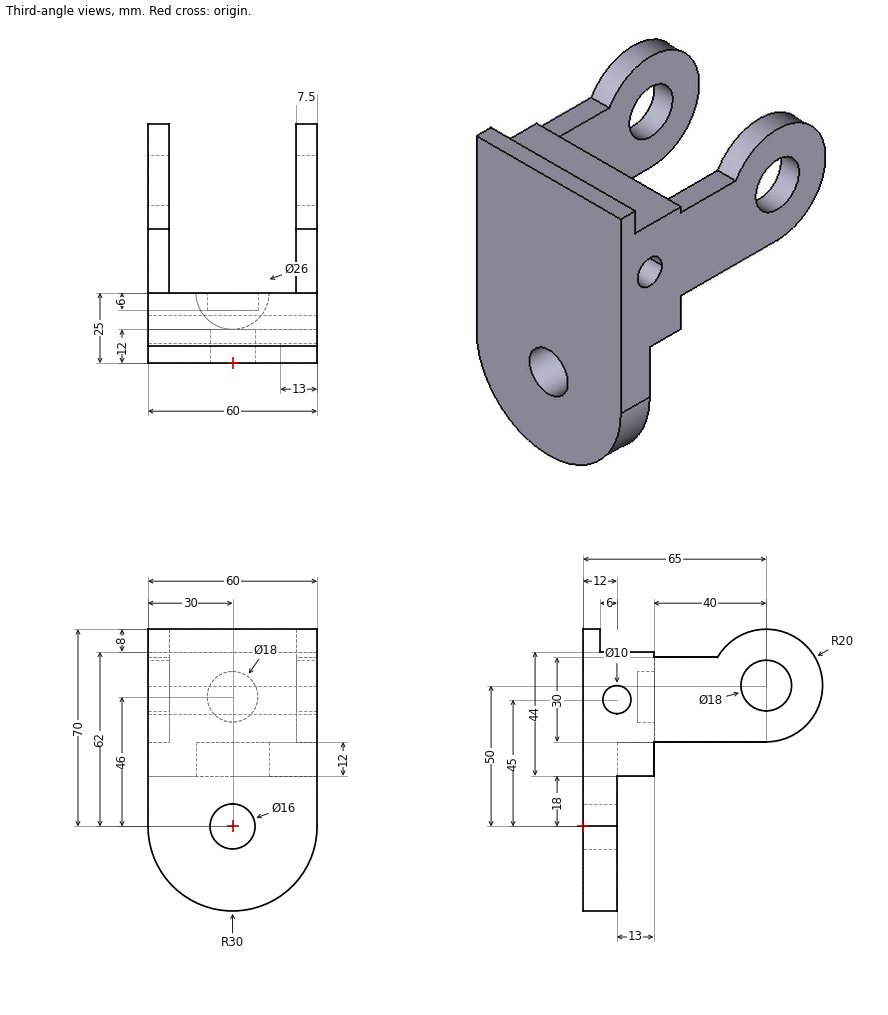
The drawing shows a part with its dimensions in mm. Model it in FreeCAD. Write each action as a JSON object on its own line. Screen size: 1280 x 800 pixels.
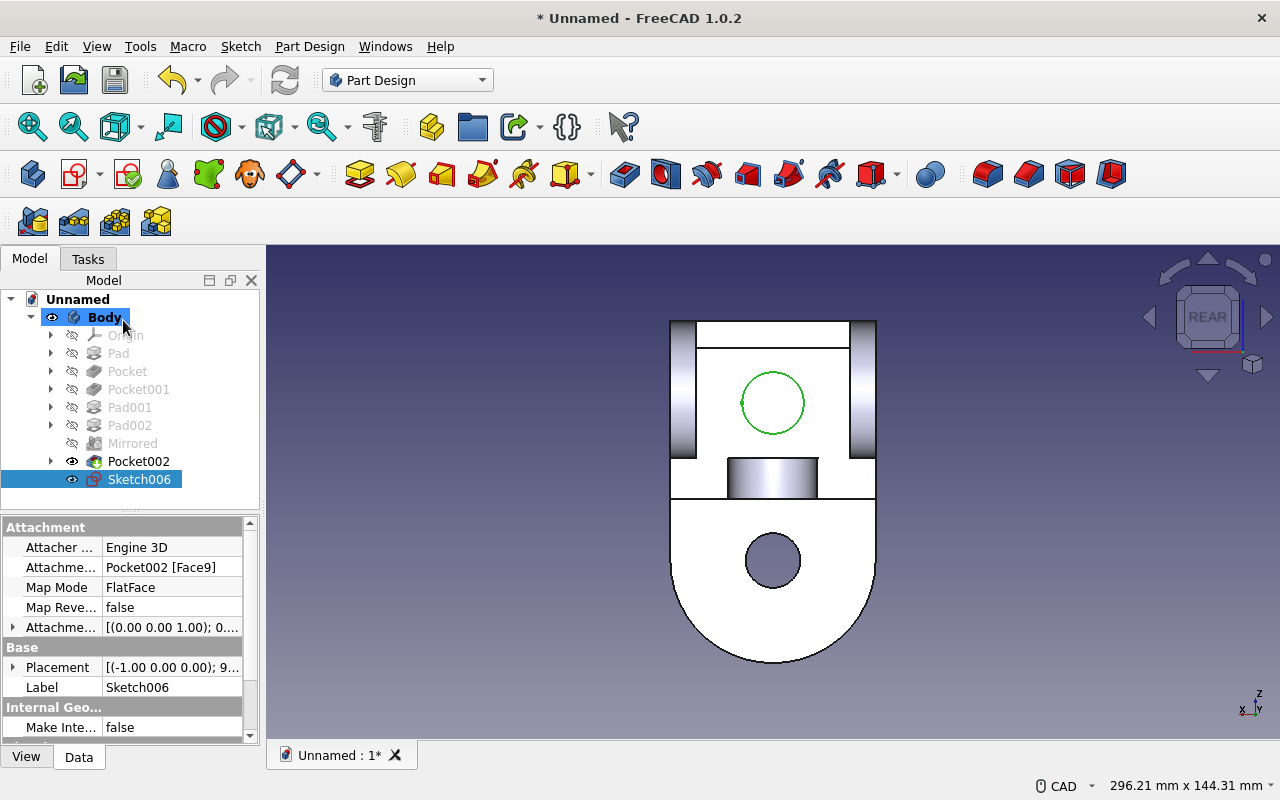
{"action": "left_click", "coordinate": [625, 174]}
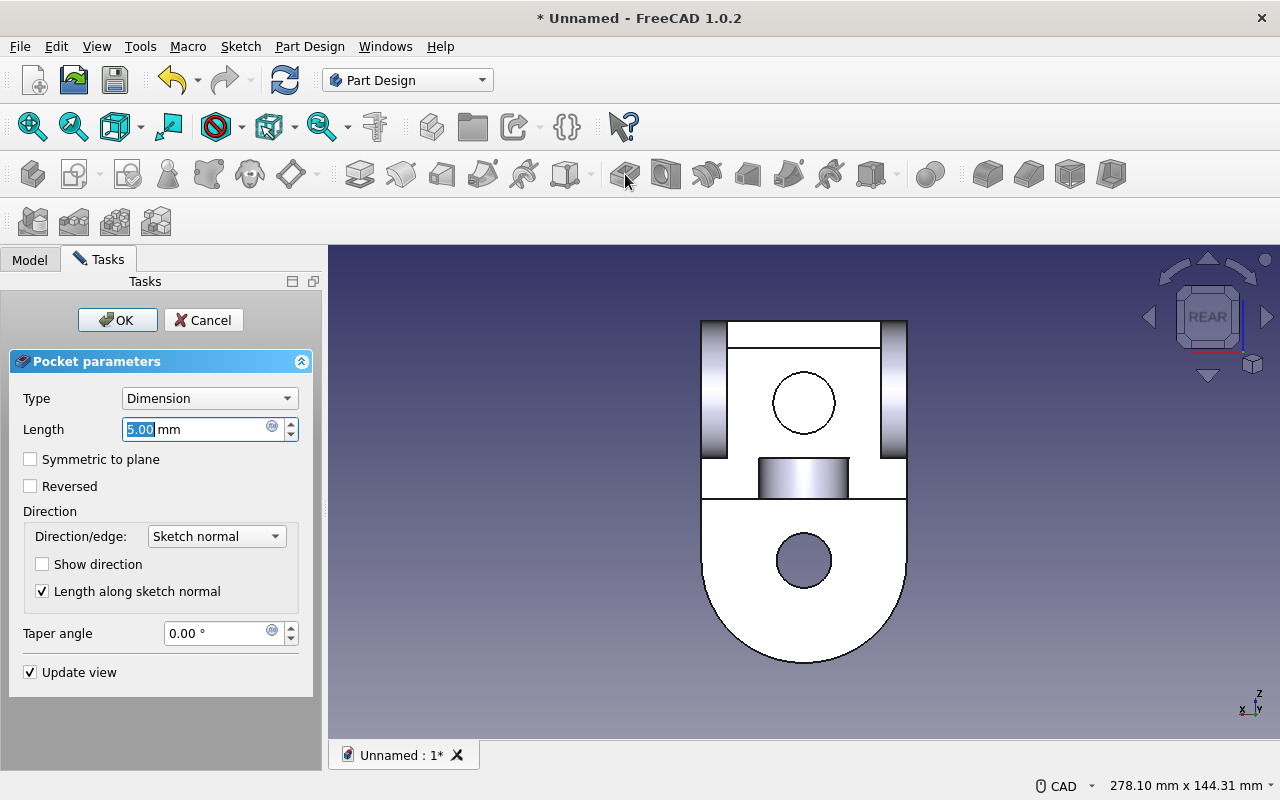
{"action": "type", "text": "6"}
{"action": "key", "text": "Tab"}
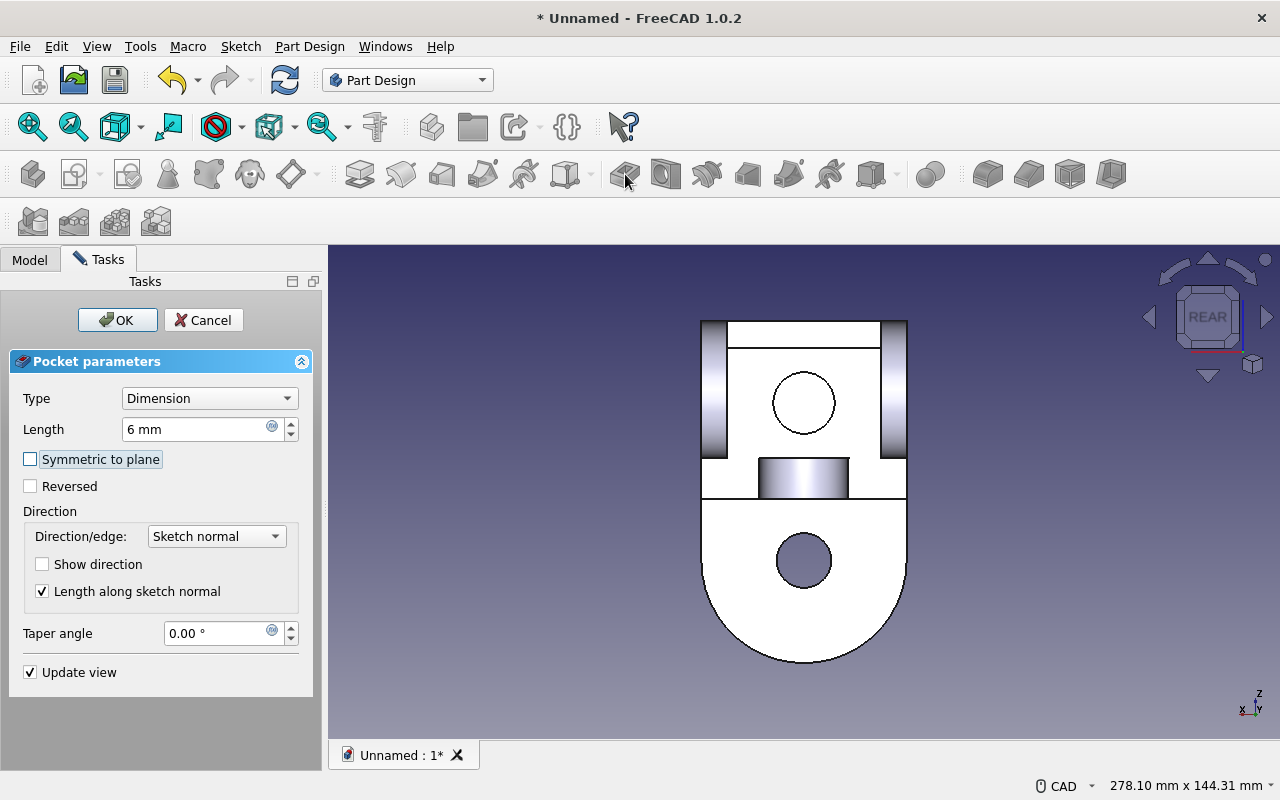
{"action": "left_click", "coordinate": [118, 320]}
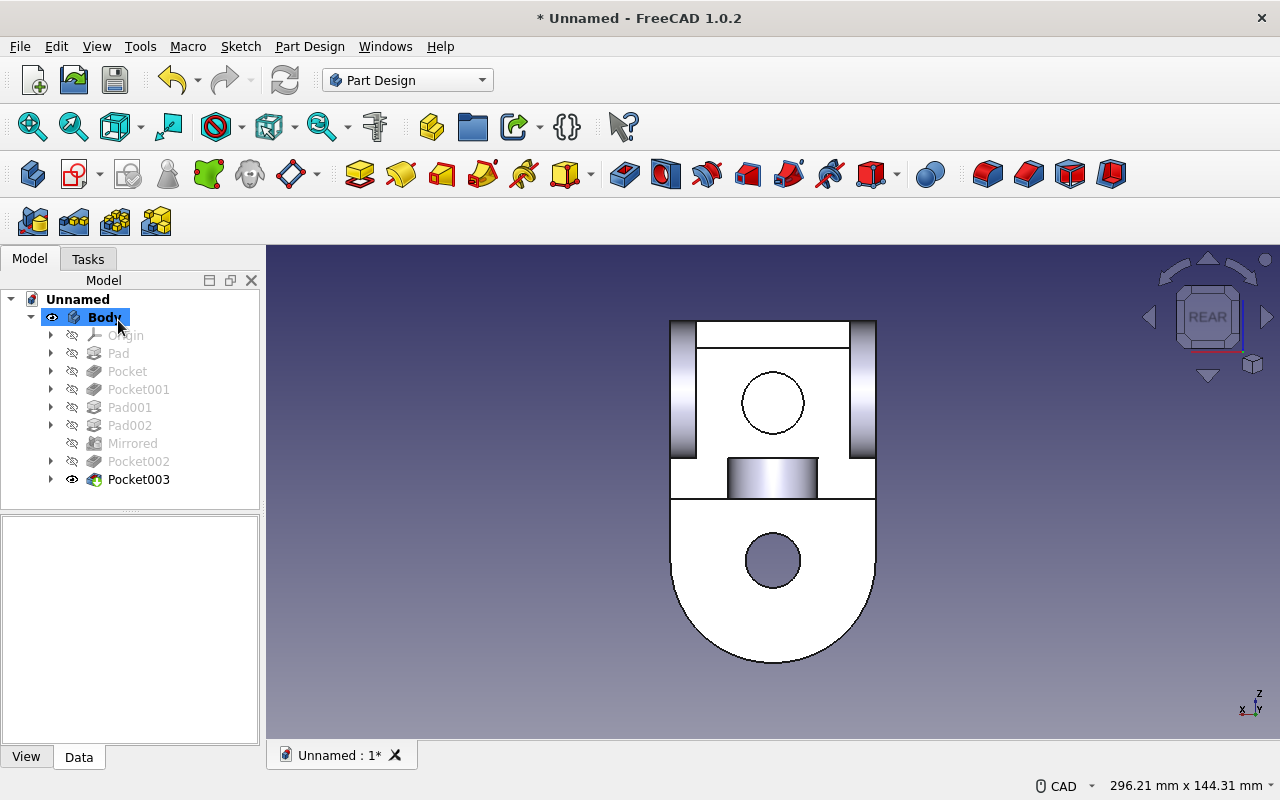
{"action": "key", "text": "0"}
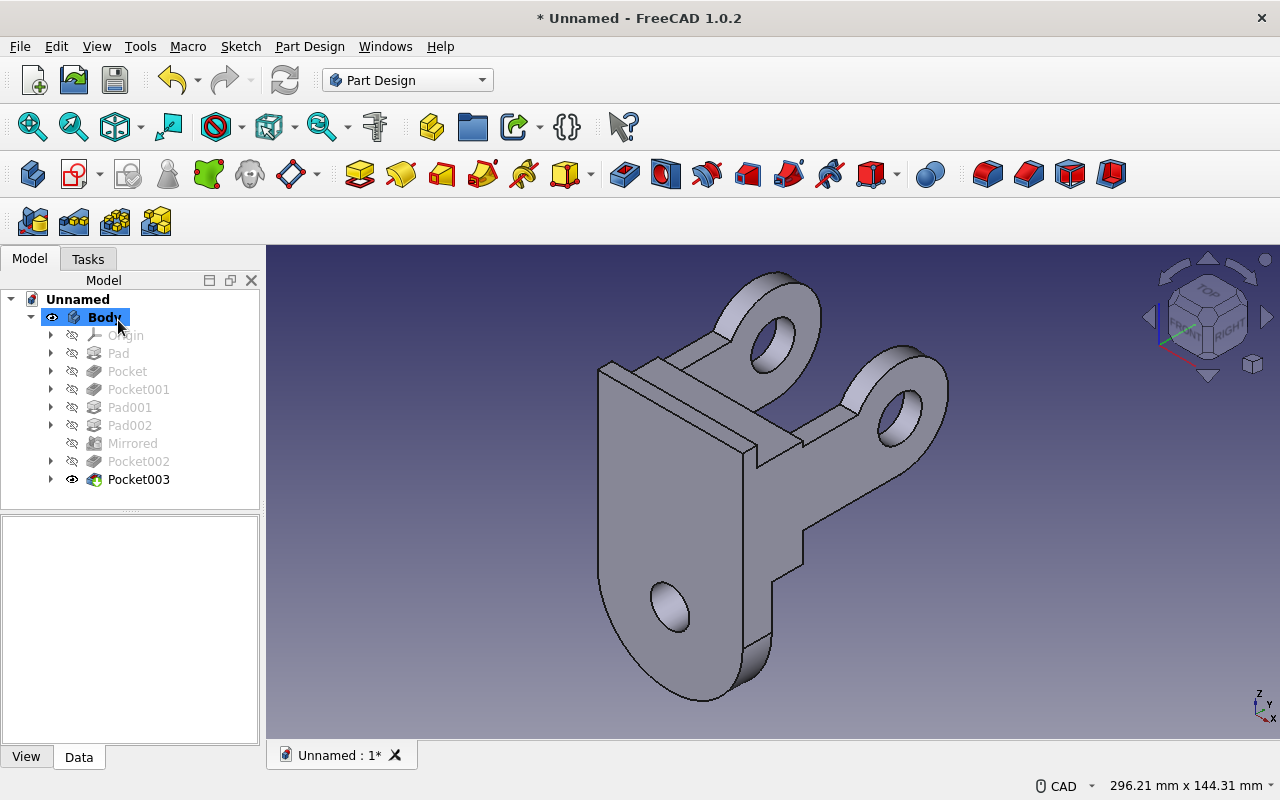
{"action": "left_click", "coordinate": [787, 497]}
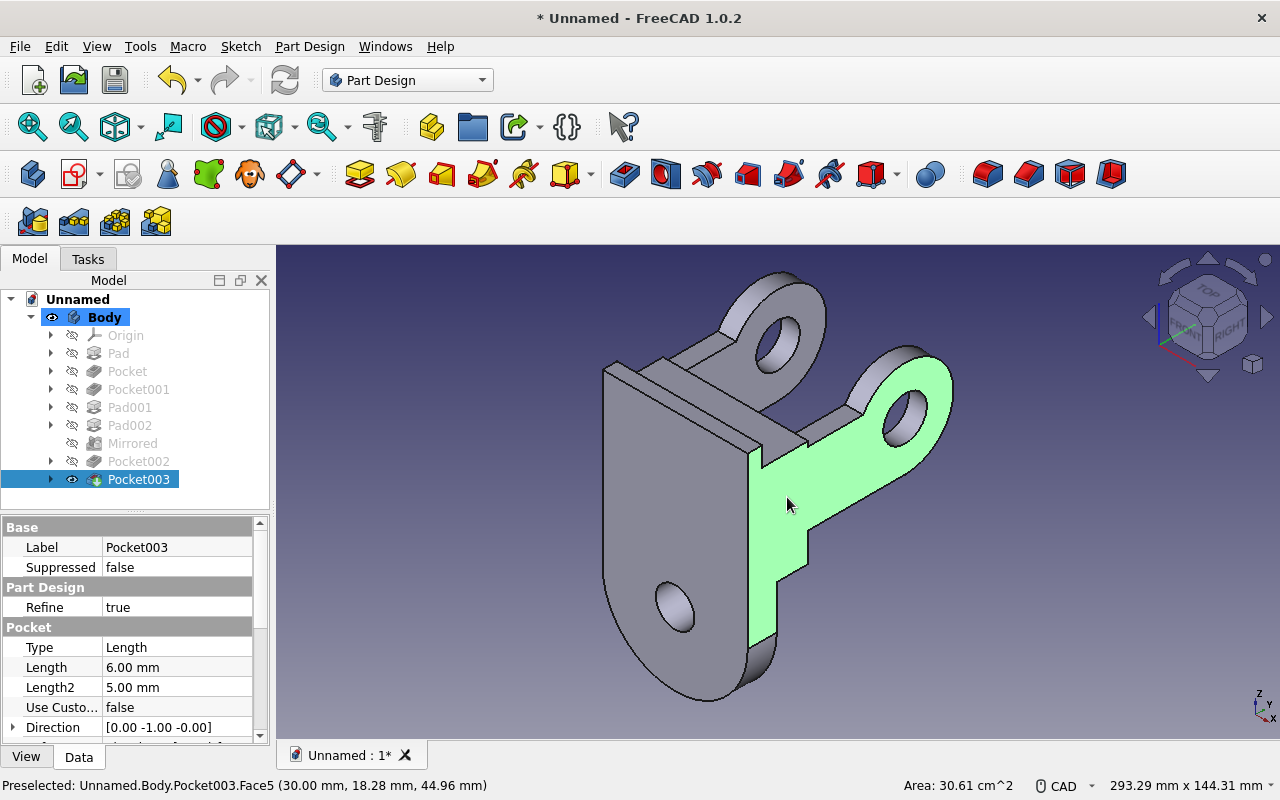
{"action": "left_click", "coordinate": [74, 174]}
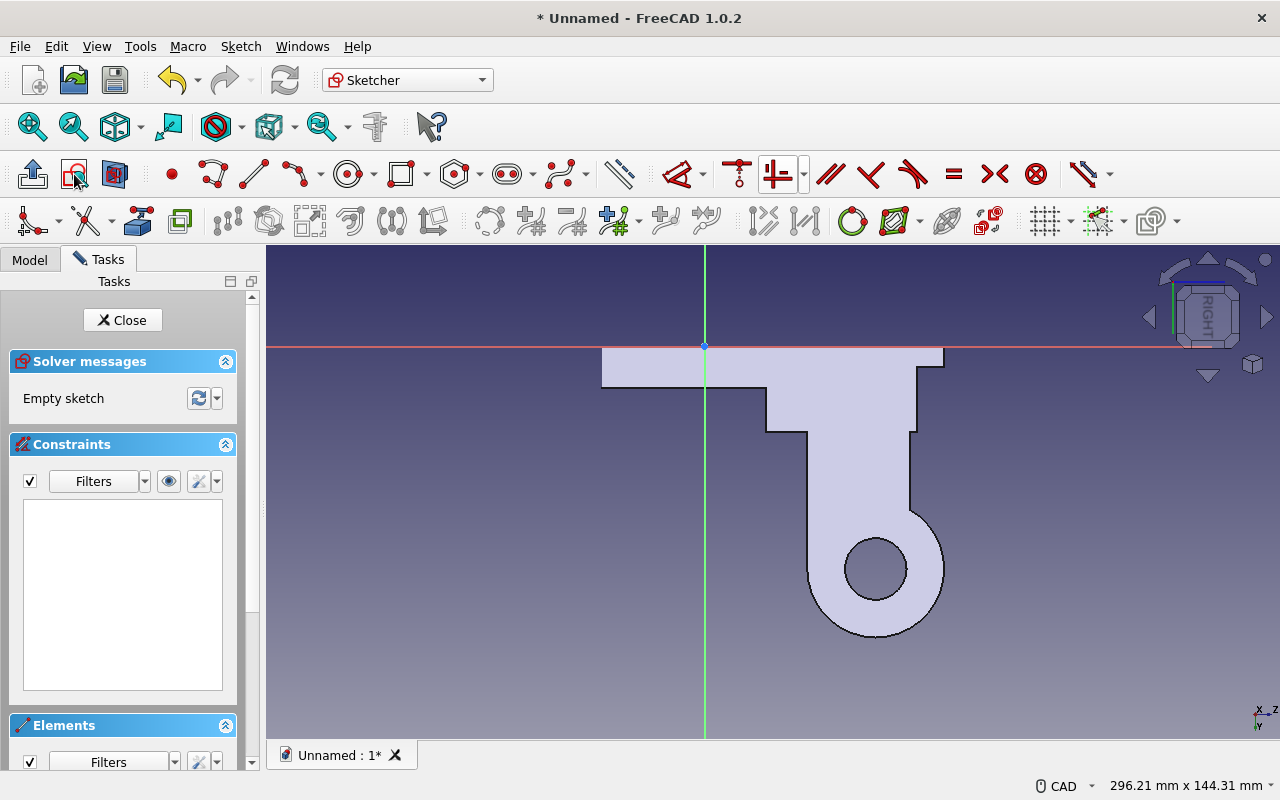
{"action": "scroll", "coordinate": [878, 375], "scroll_direction": "up", "scroll_amount": 11}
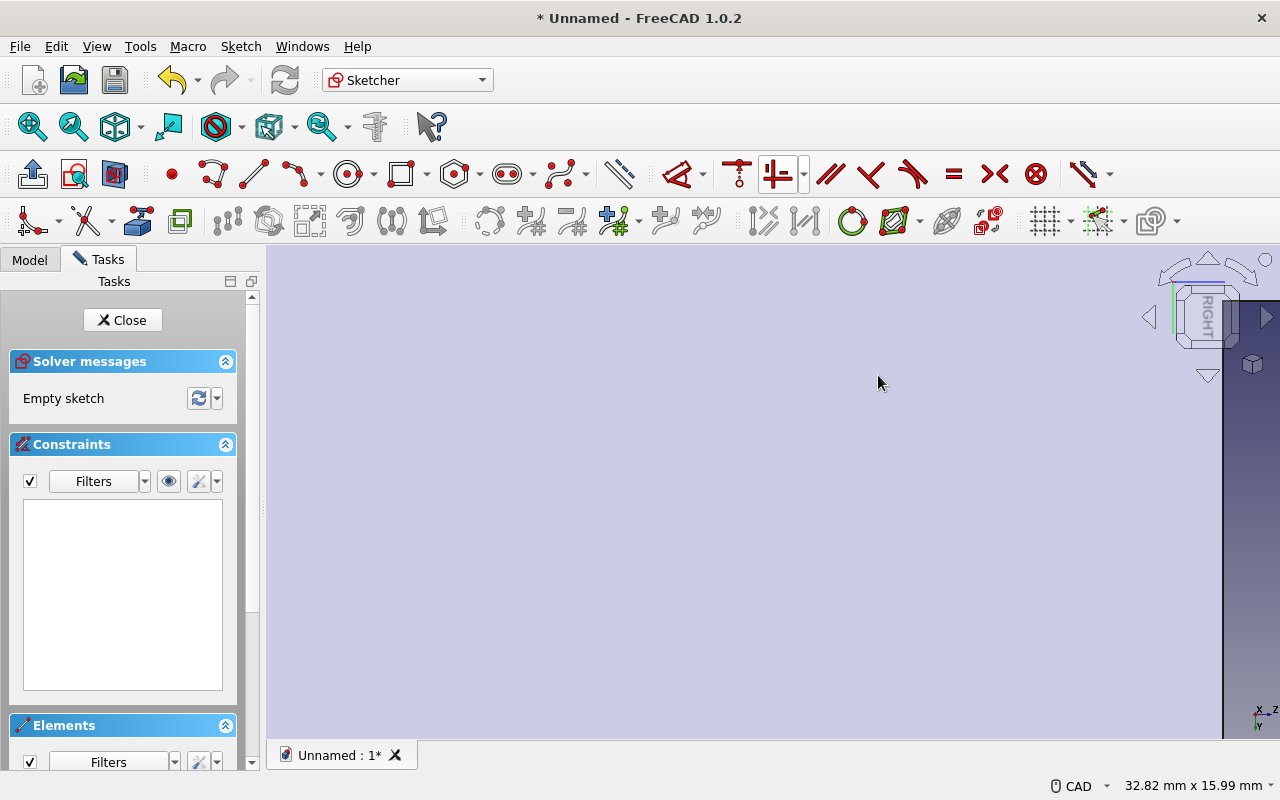
{"action": "left_click", "coordinate": [348, 174]}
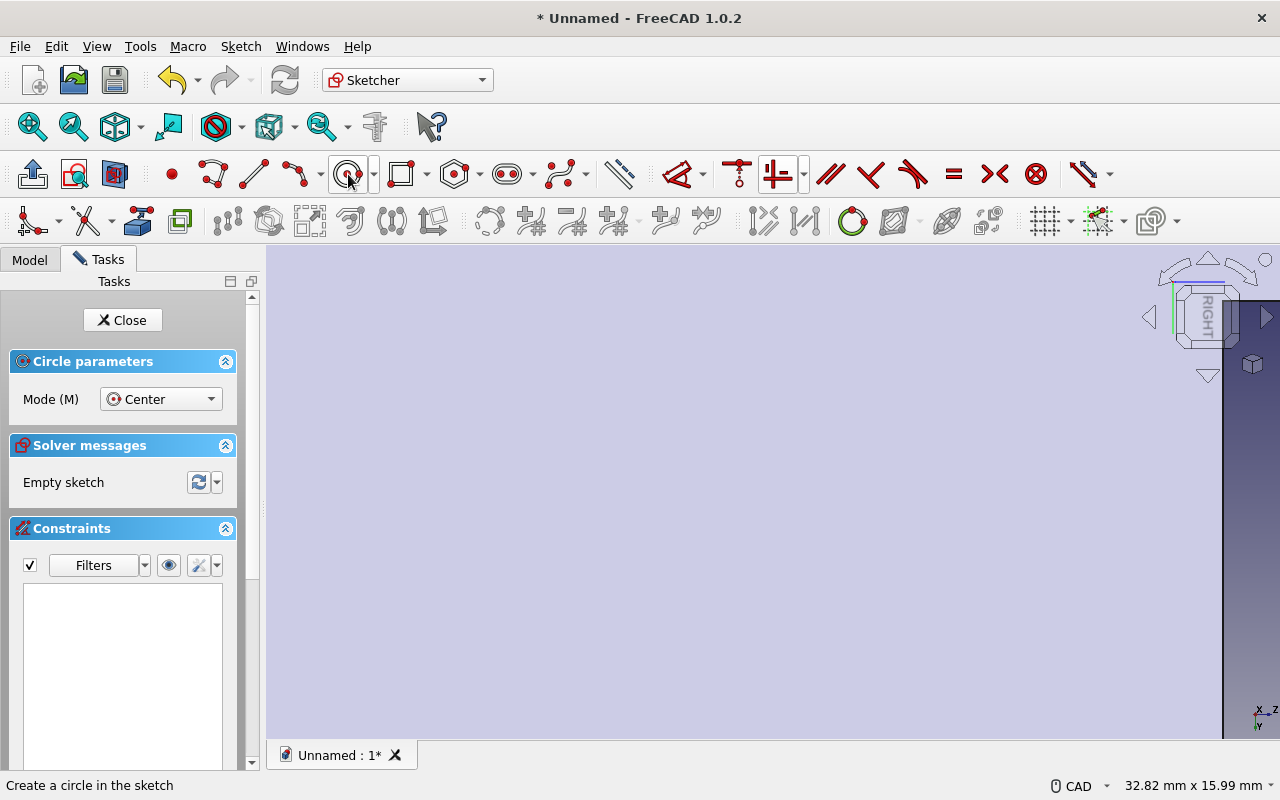
{"action": "left_click", "coordinate": [698, 487]}
{"action": "left_click", "coordinate": [807, 377]}
{"action": "key", "text": "Escape"}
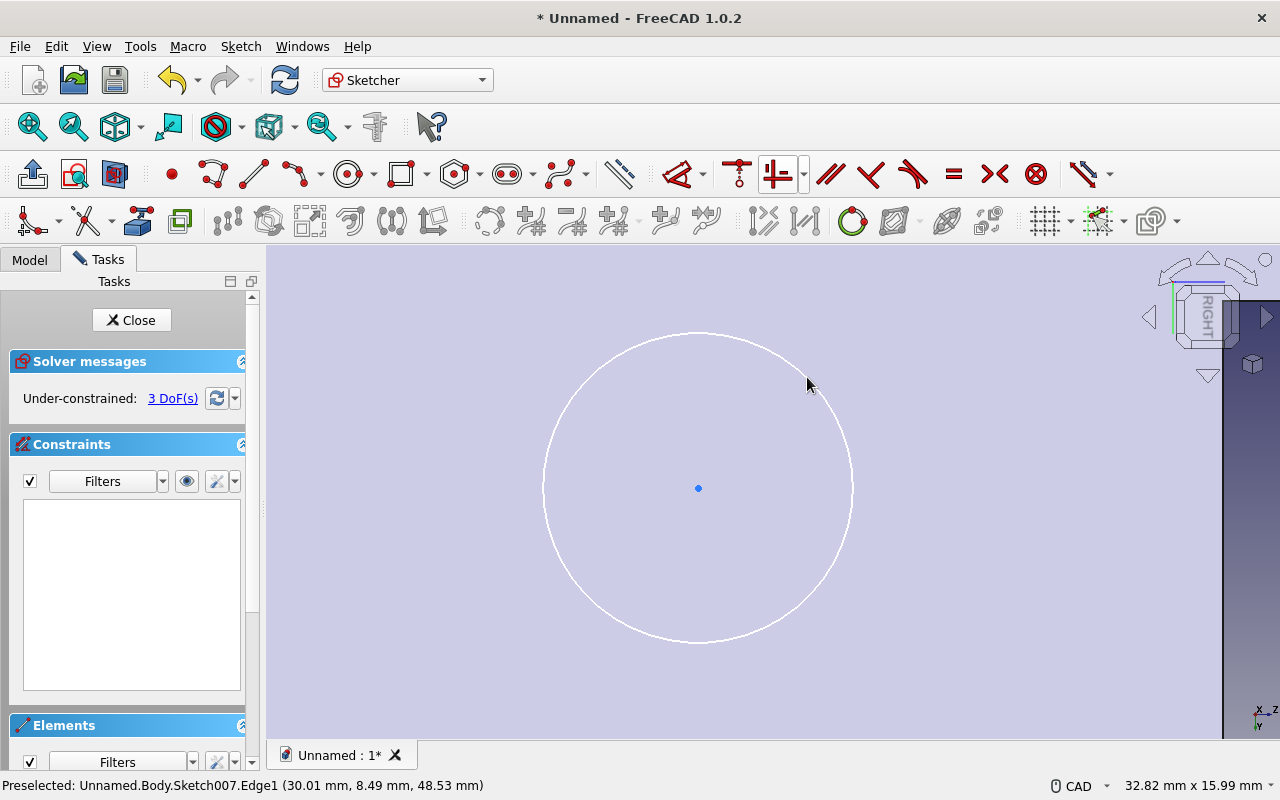
{"action": "left_click", "coordinate": [676, 174]}